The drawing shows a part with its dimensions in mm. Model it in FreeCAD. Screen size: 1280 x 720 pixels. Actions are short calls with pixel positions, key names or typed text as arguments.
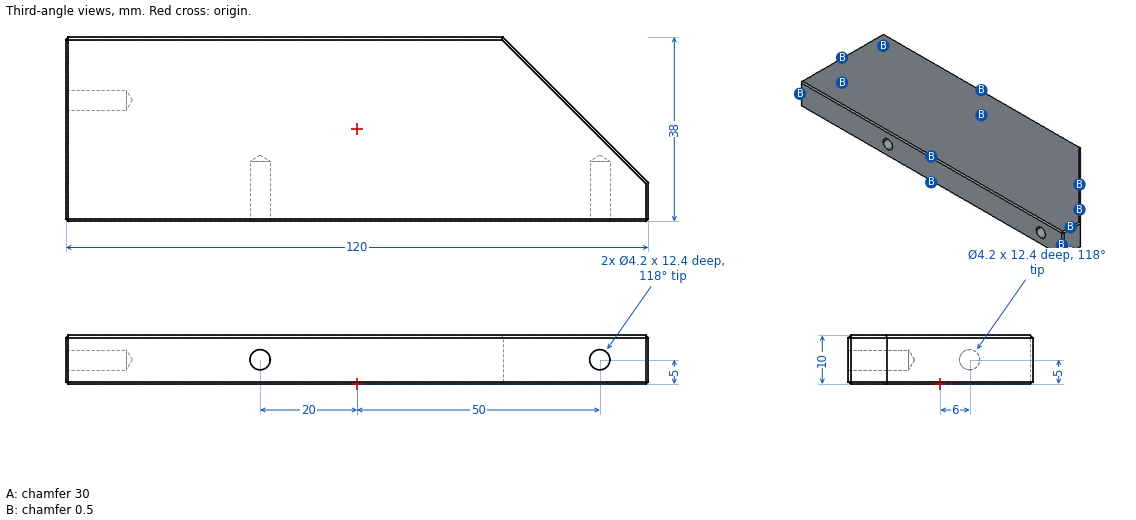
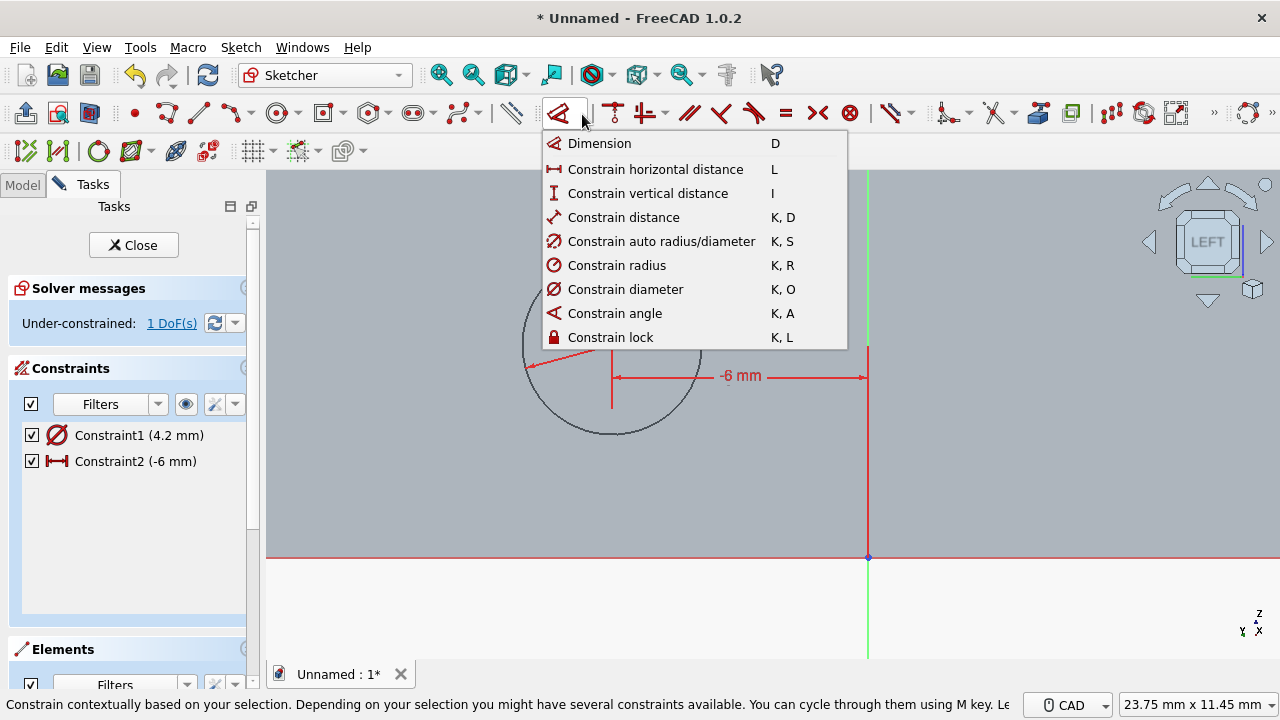
click(695, 193)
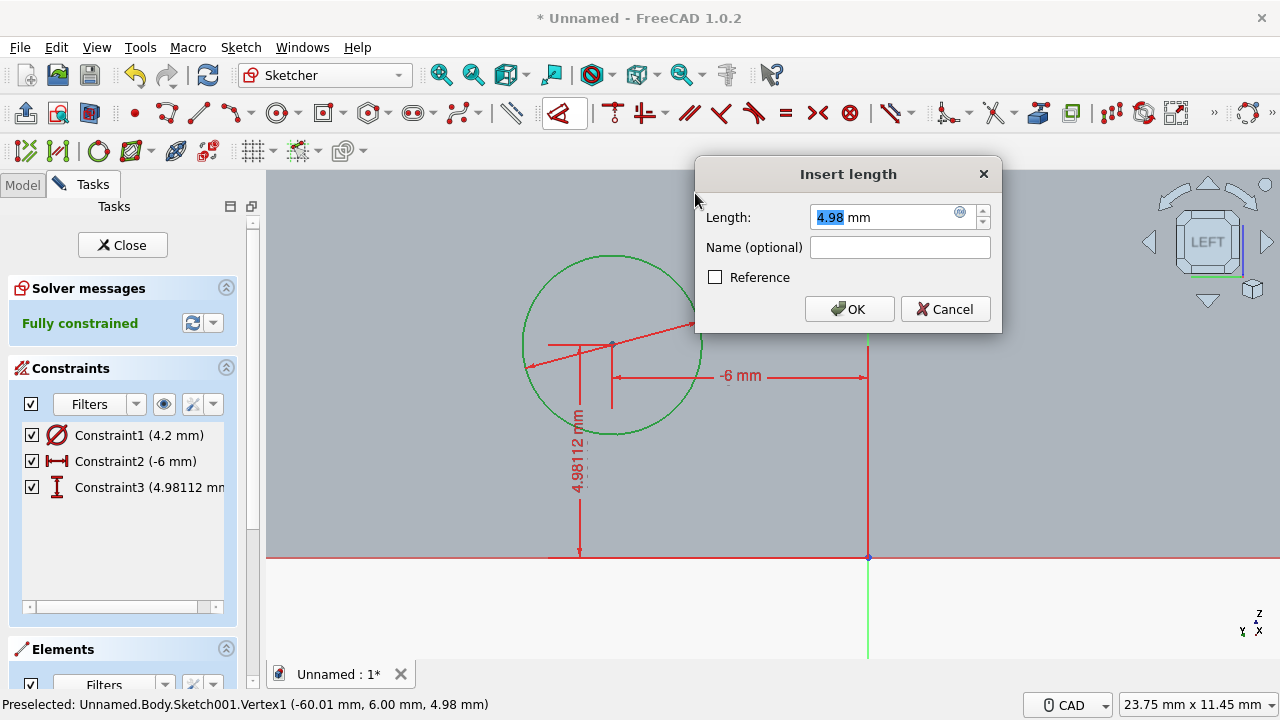
text(5)
key(Return)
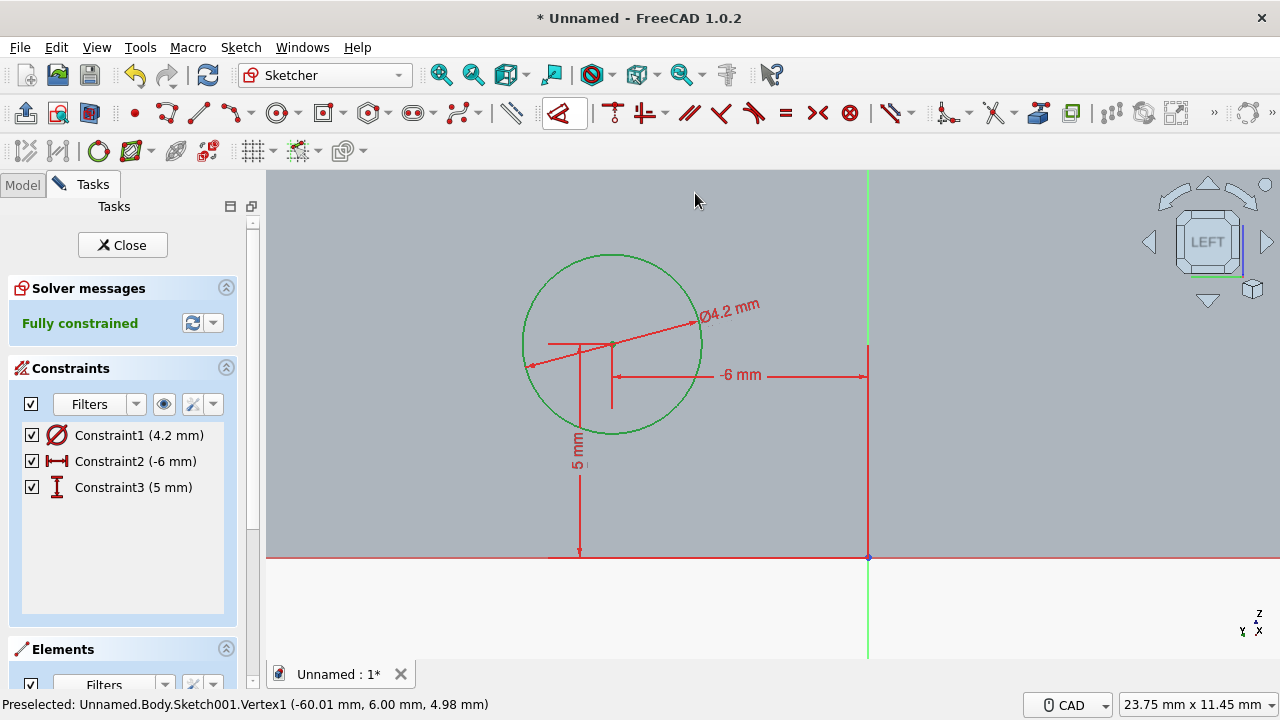
click(123, 245)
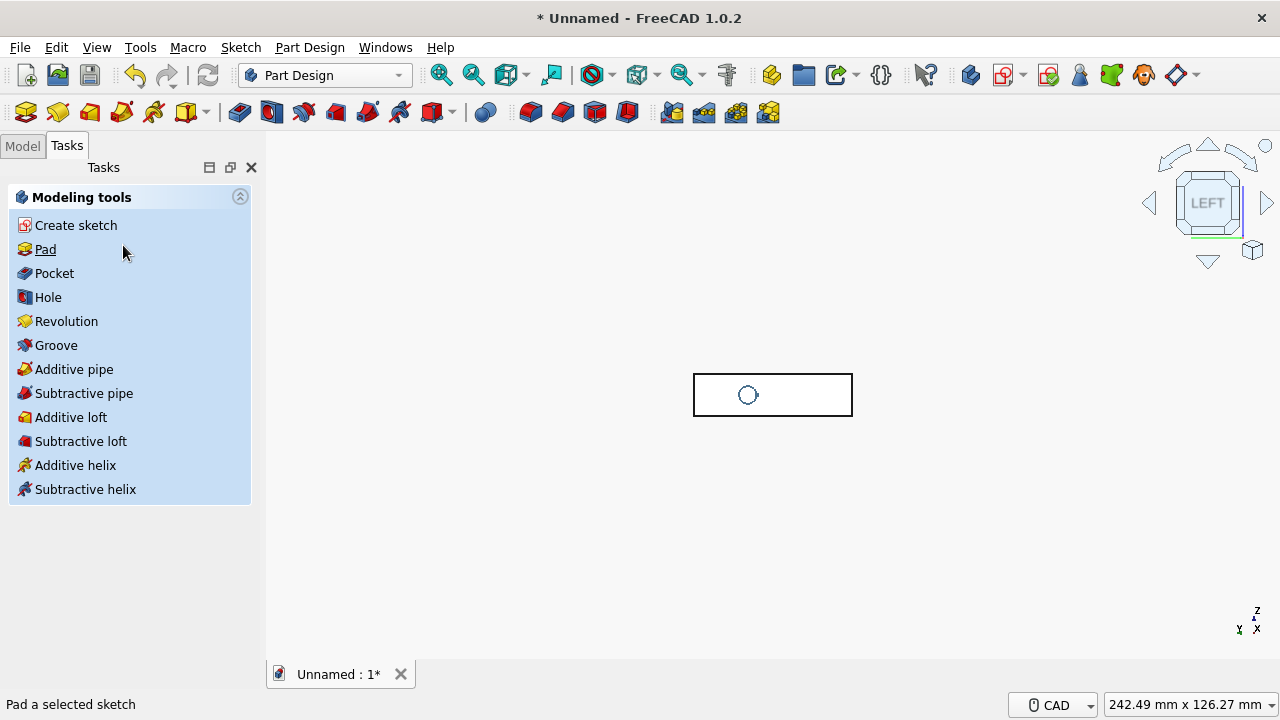
click(272, 112)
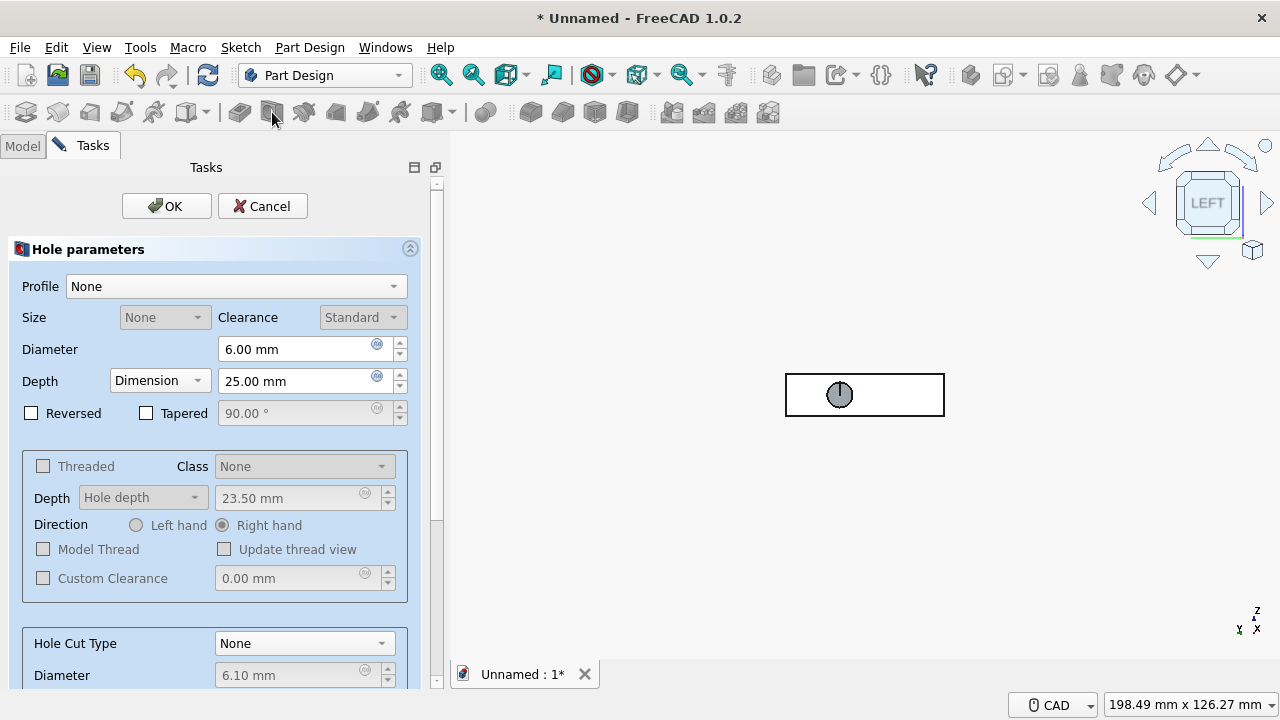
triple_click(305, 349)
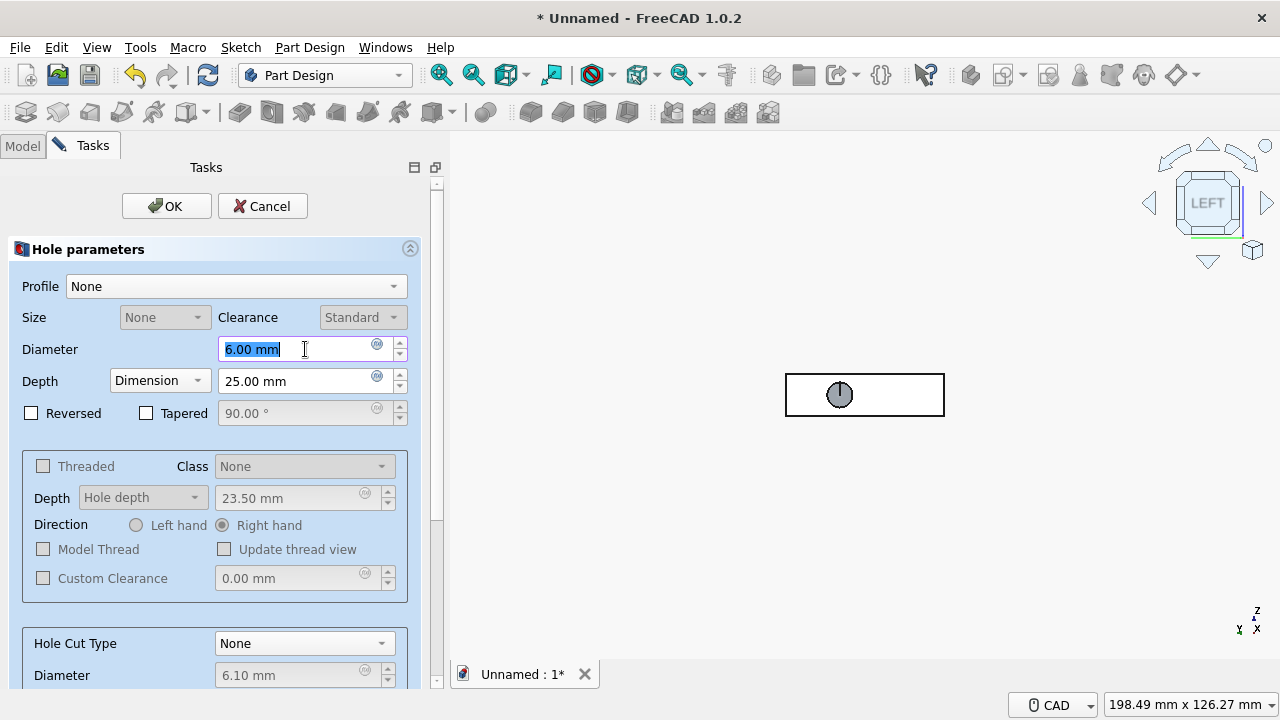
text(4.2)
key(Tab)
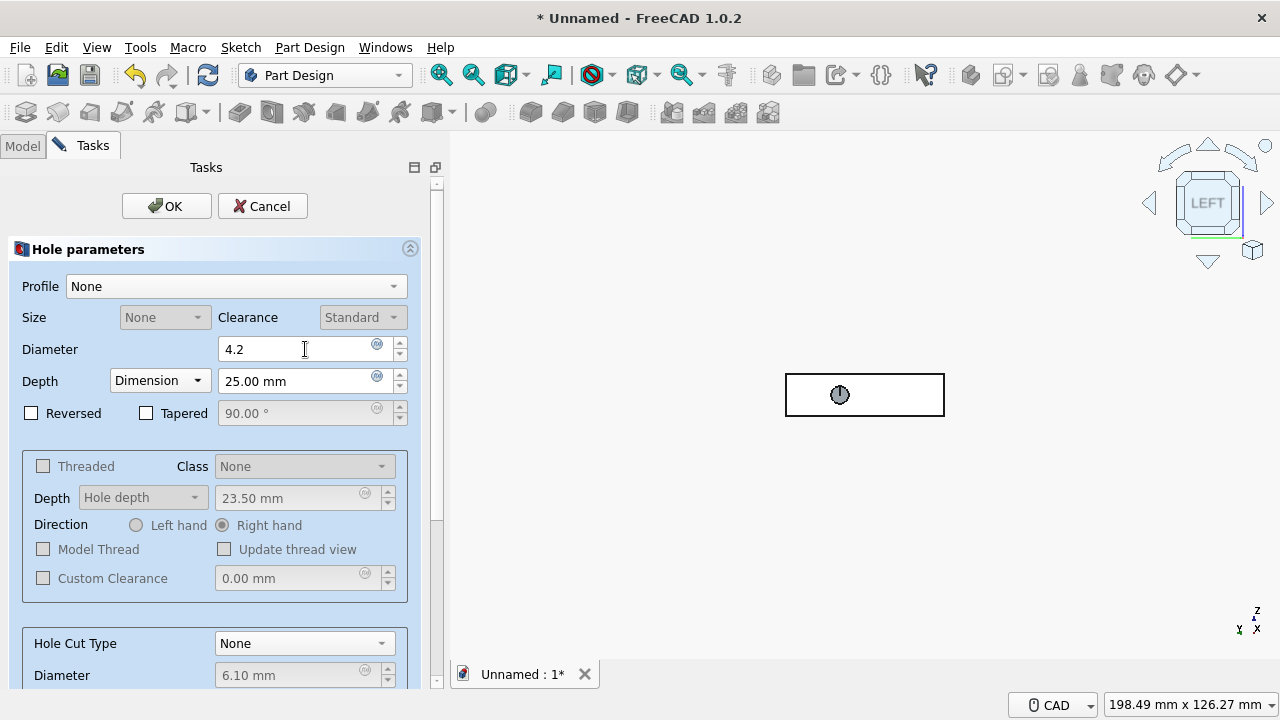
triple_click(305, 381)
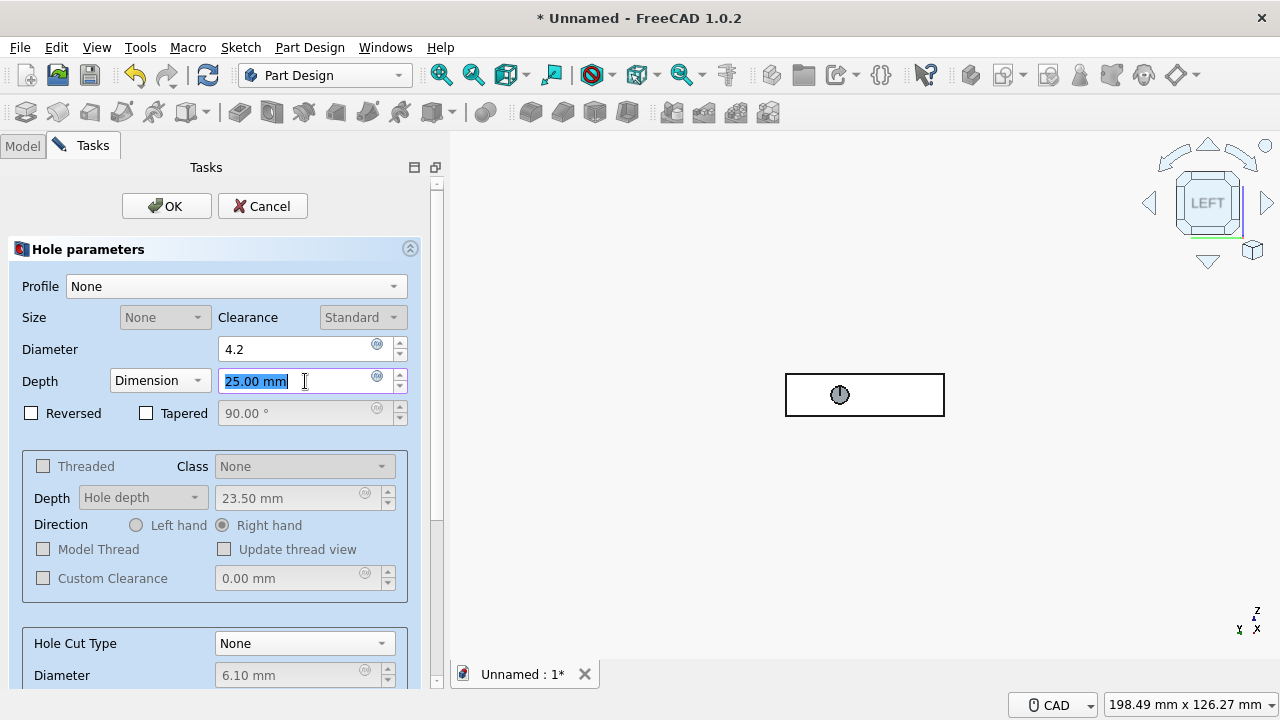
text(12.4)
key(Tab)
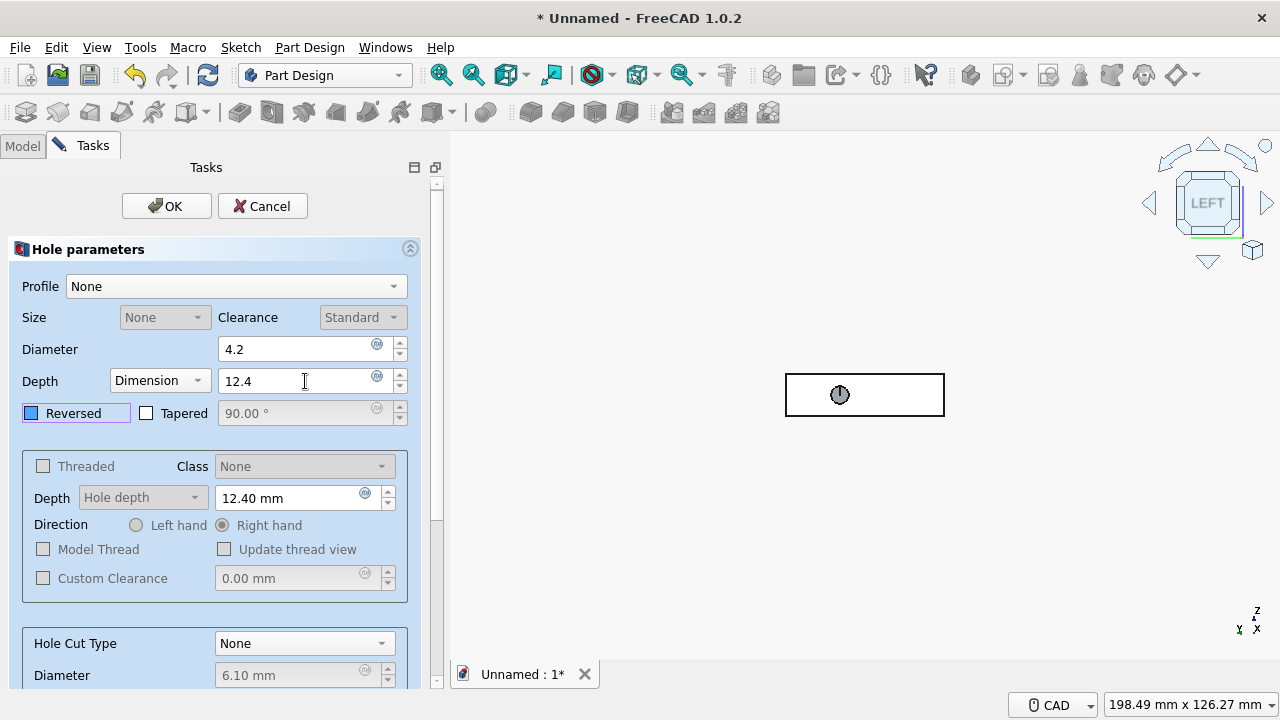
click(167, 206)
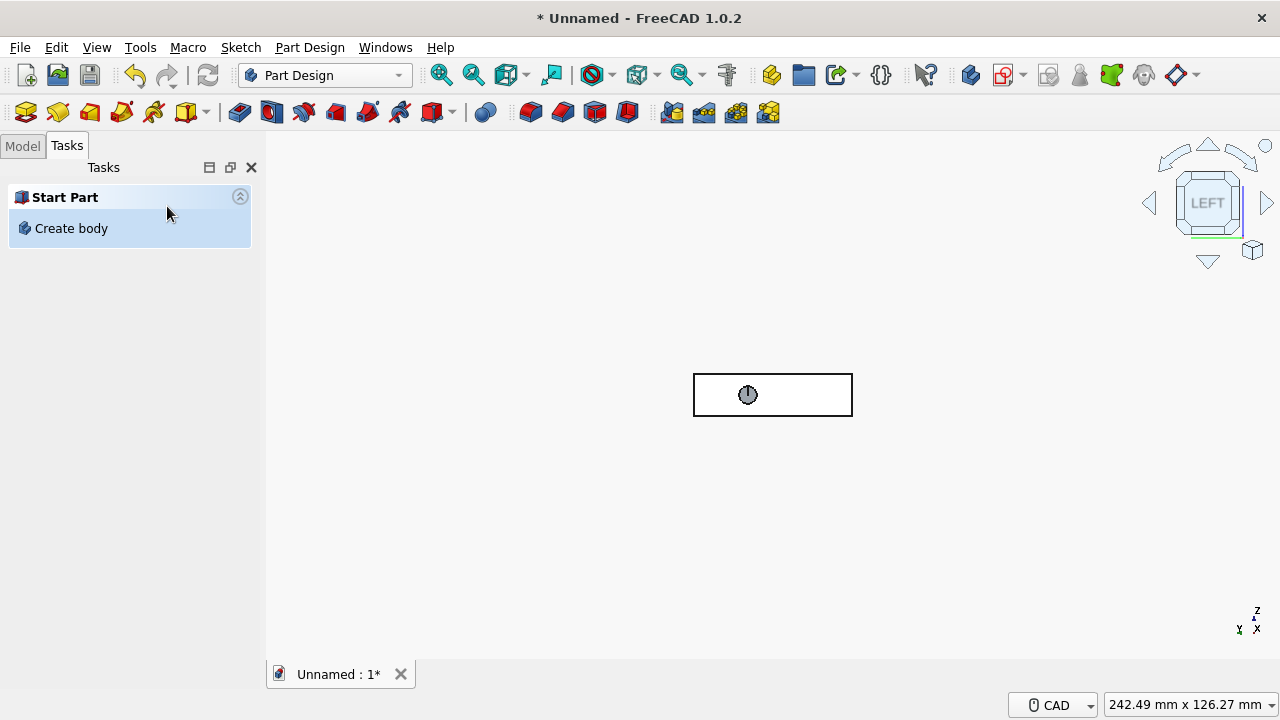
click(442, 76)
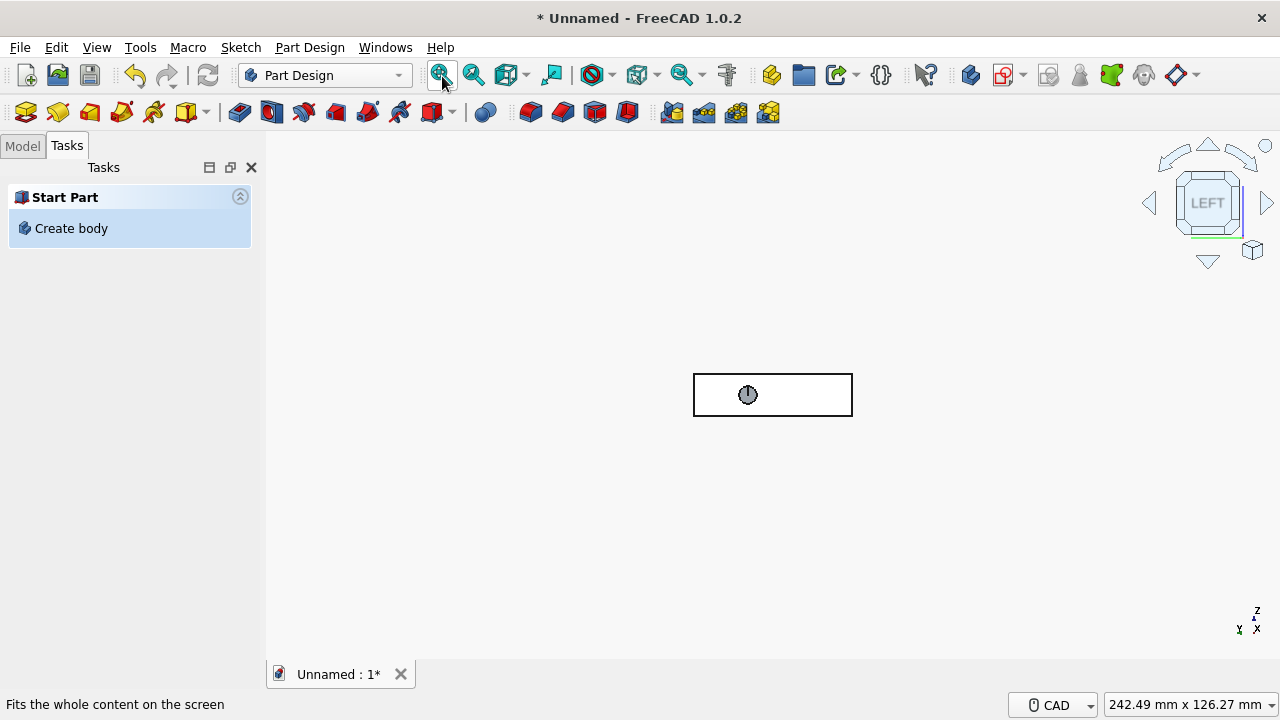
key(0)